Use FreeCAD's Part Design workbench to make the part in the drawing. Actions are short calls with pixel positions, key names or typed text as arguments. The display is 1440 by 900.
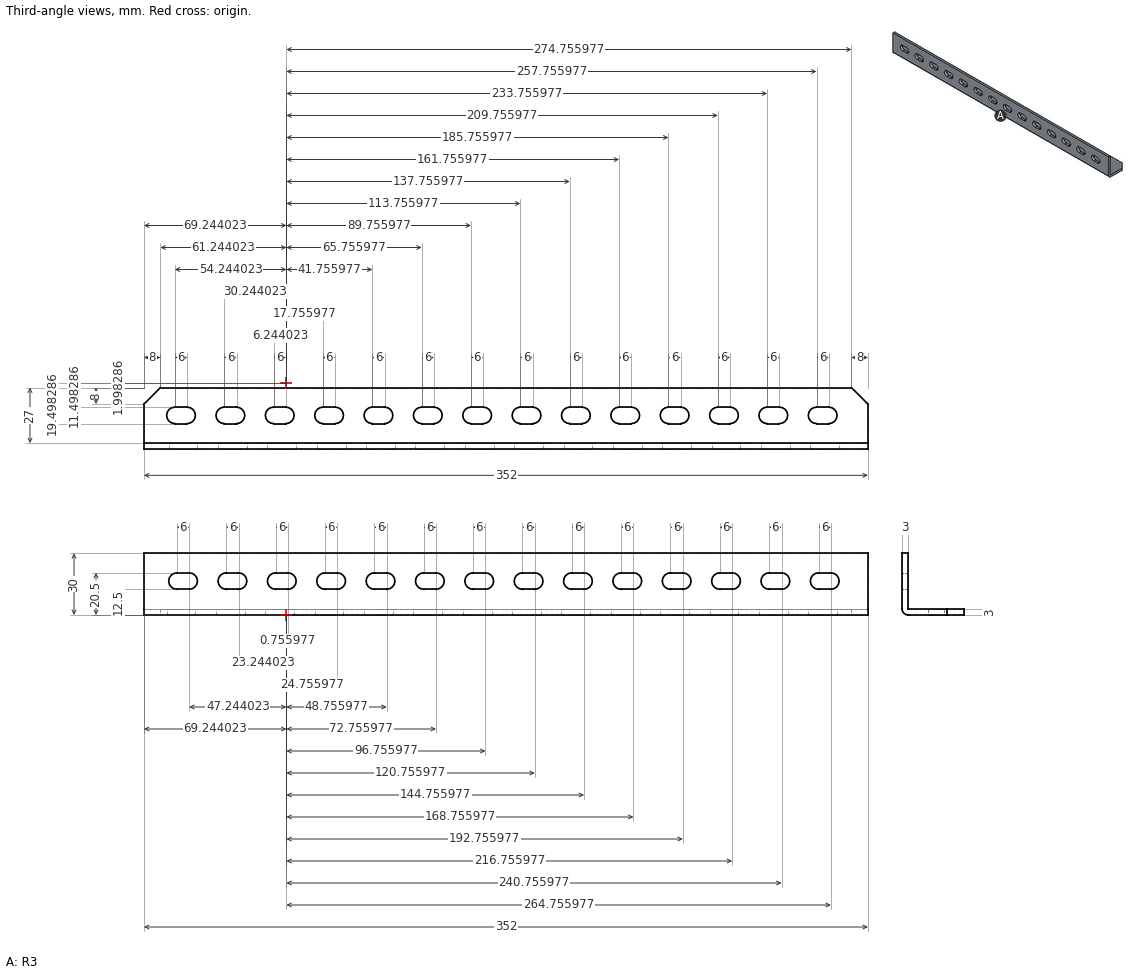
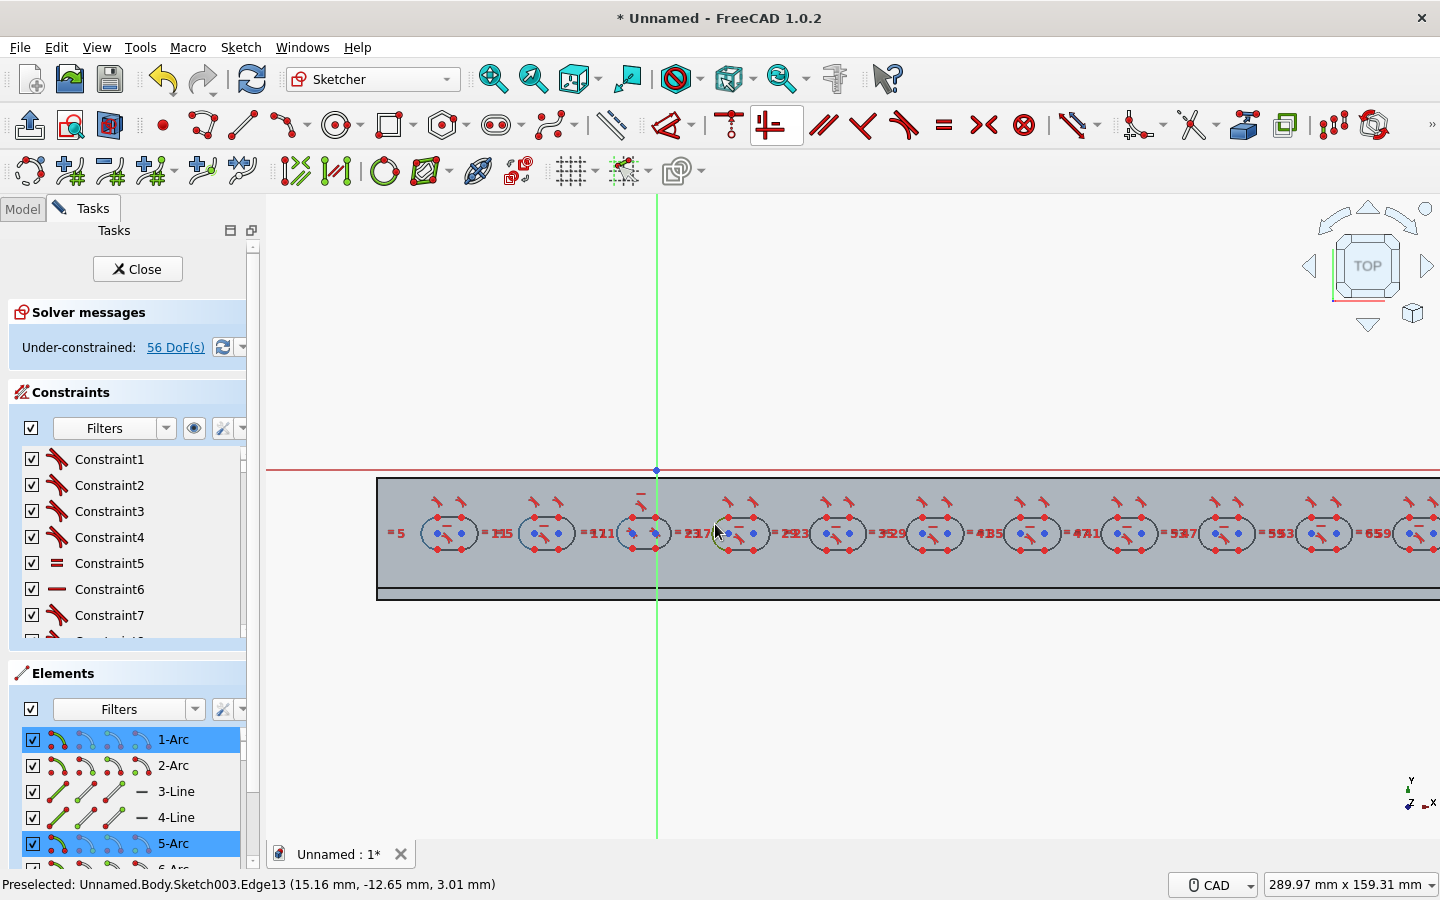
click(813, 524)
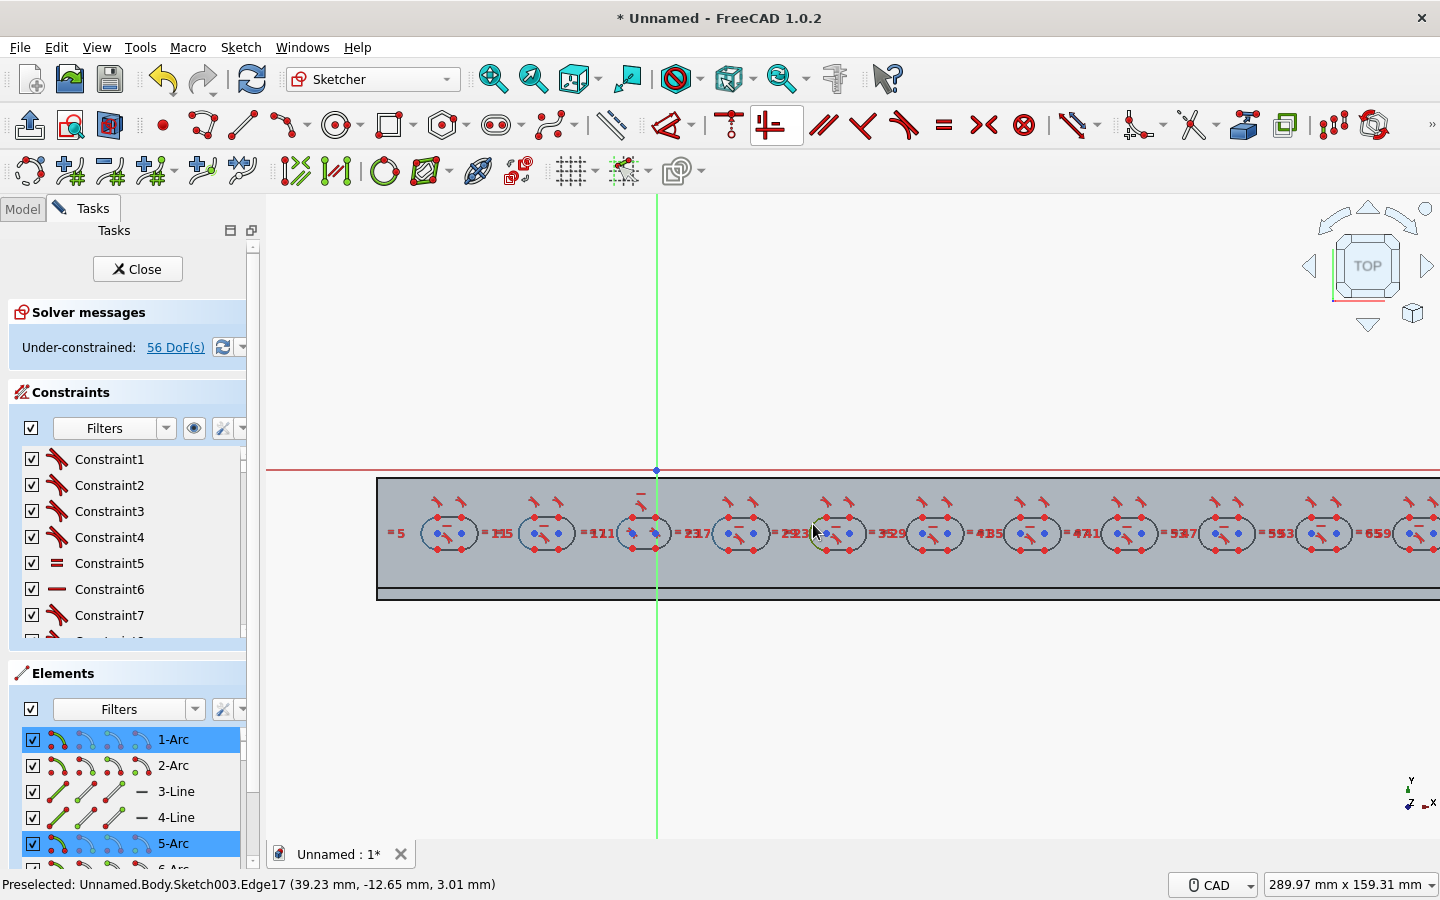
click(910, 524)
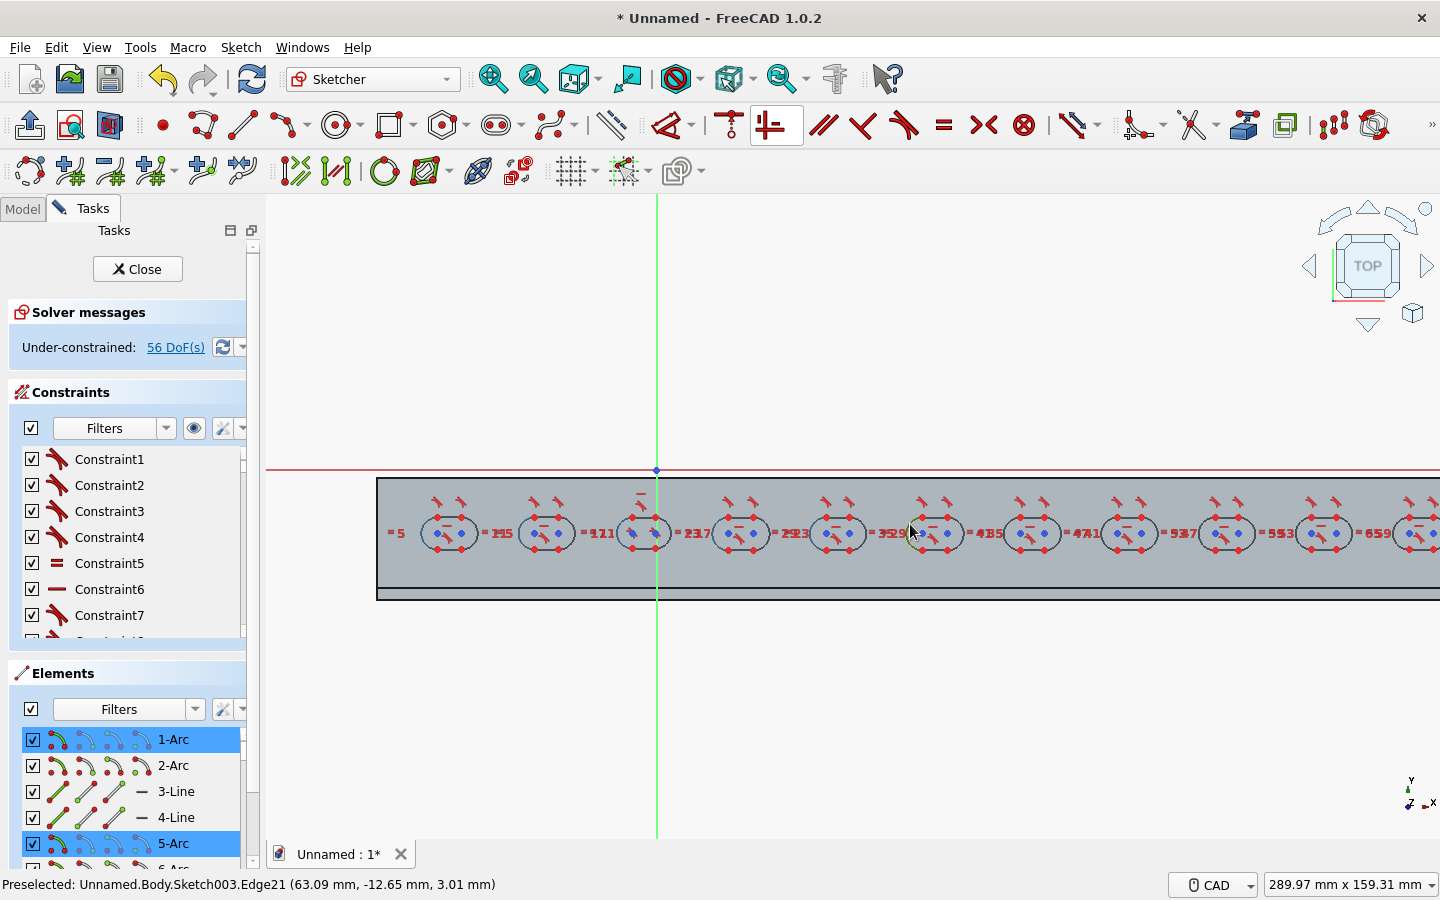
click(1007, 524)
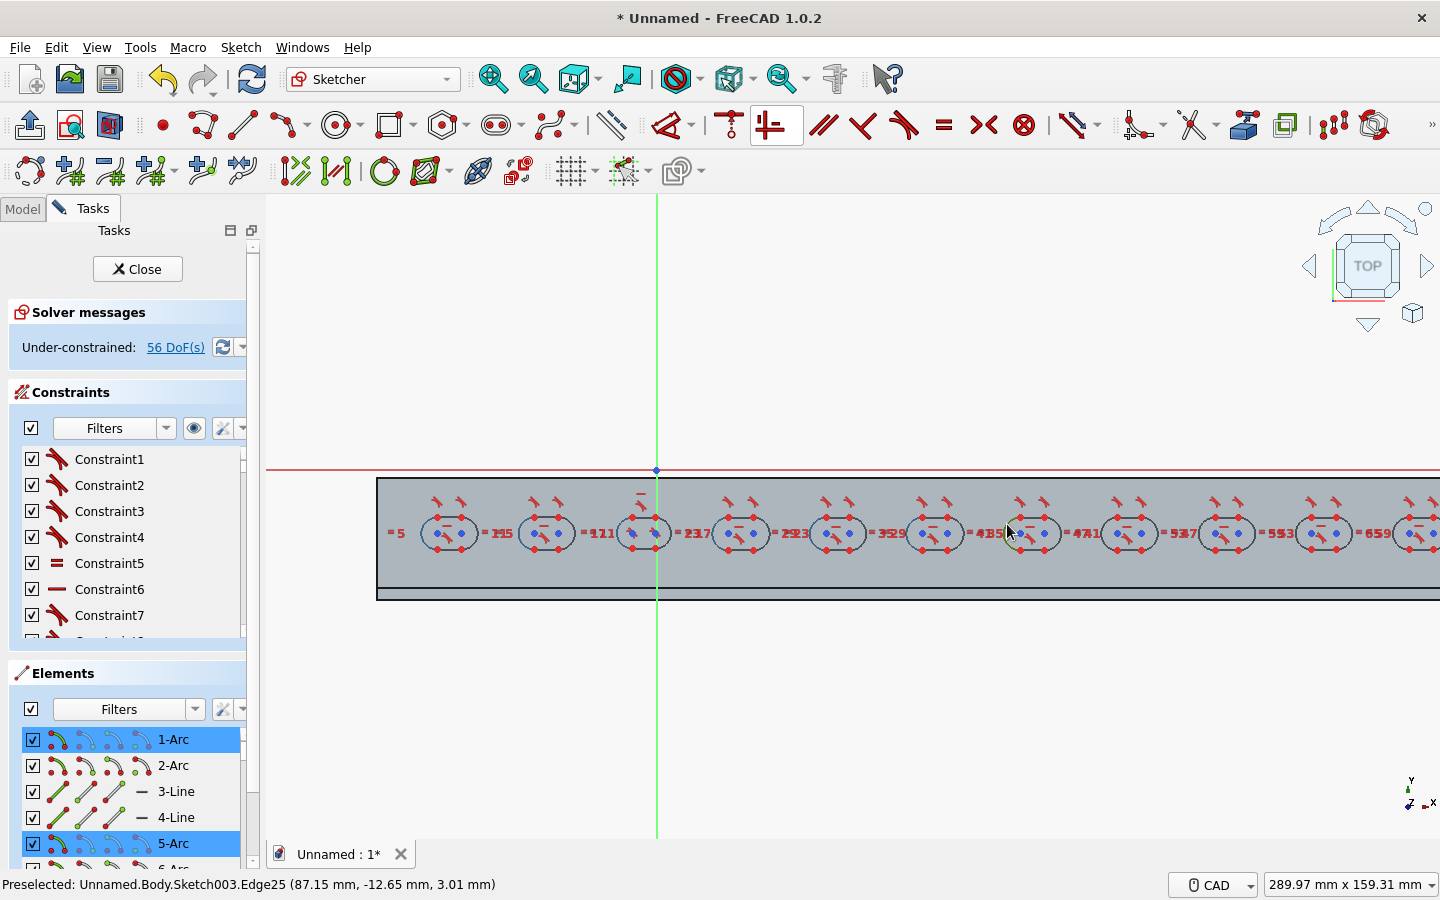
click(1104, 524)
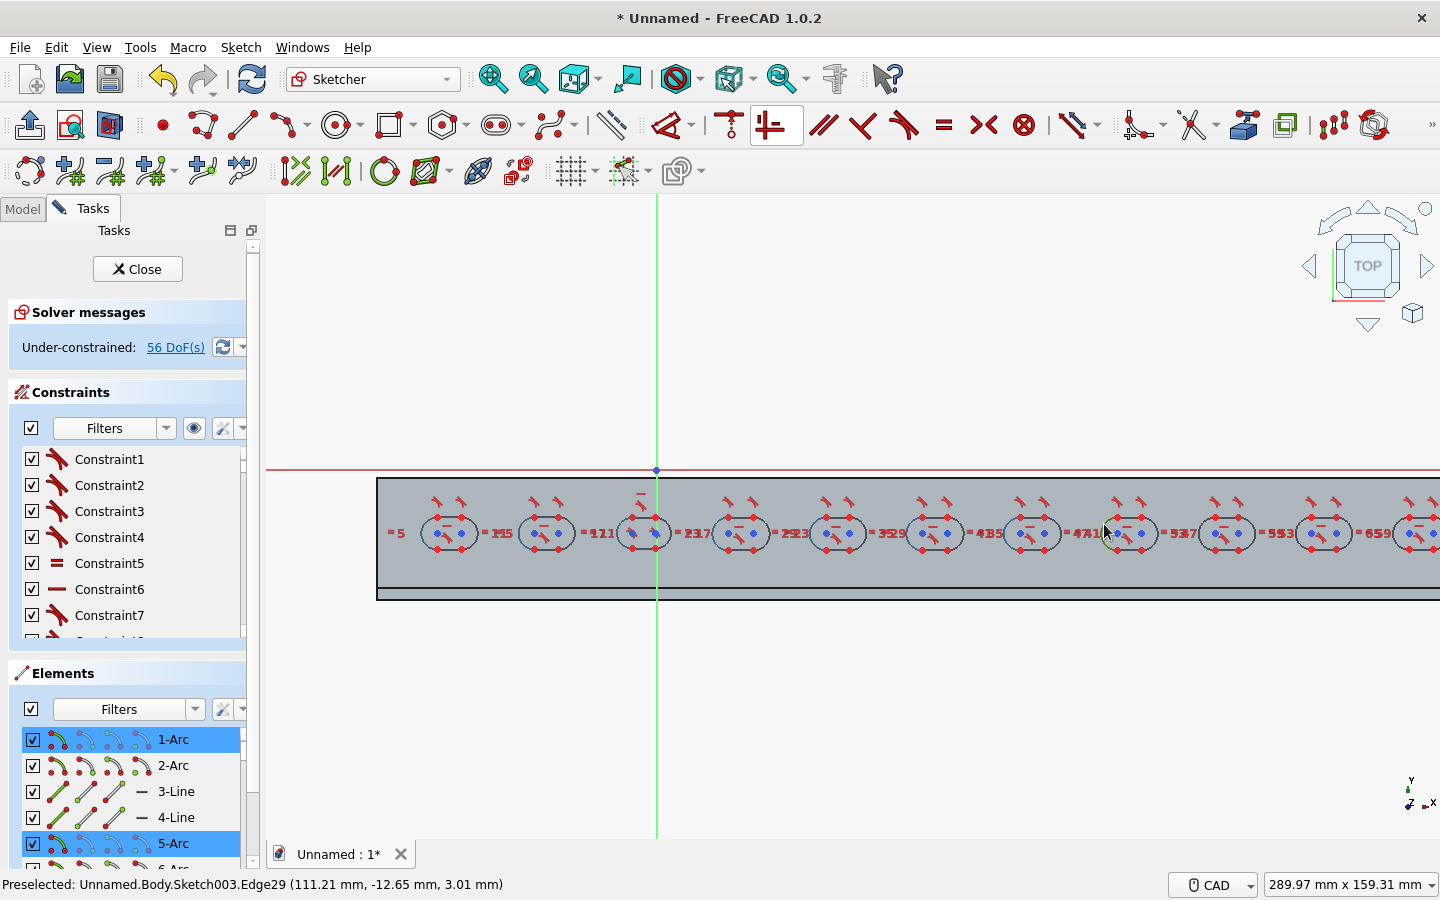
click(1202, 524)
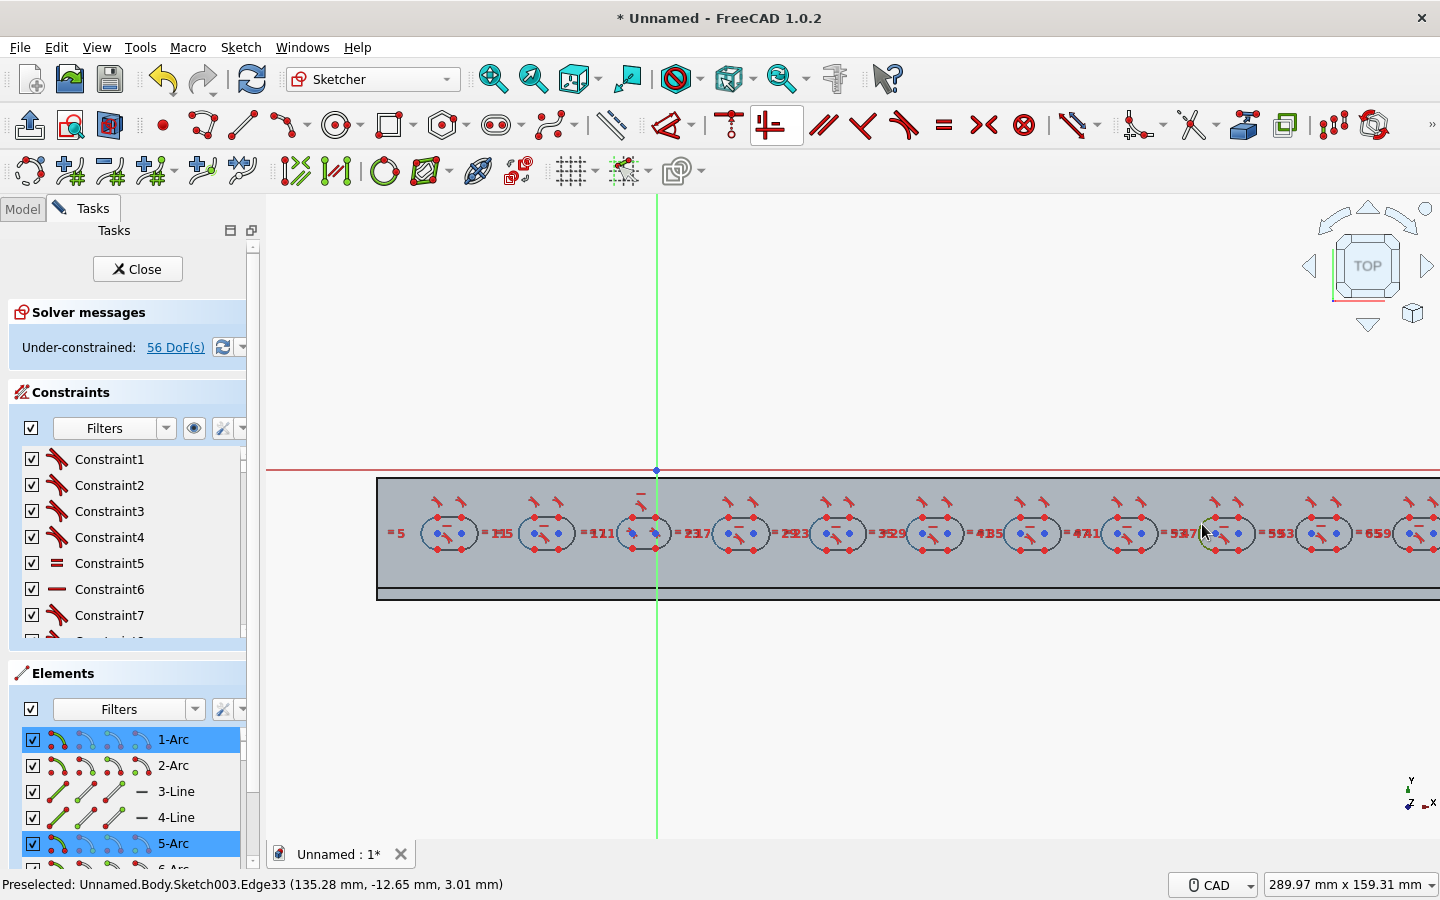
scroll(424, 525, down, 3)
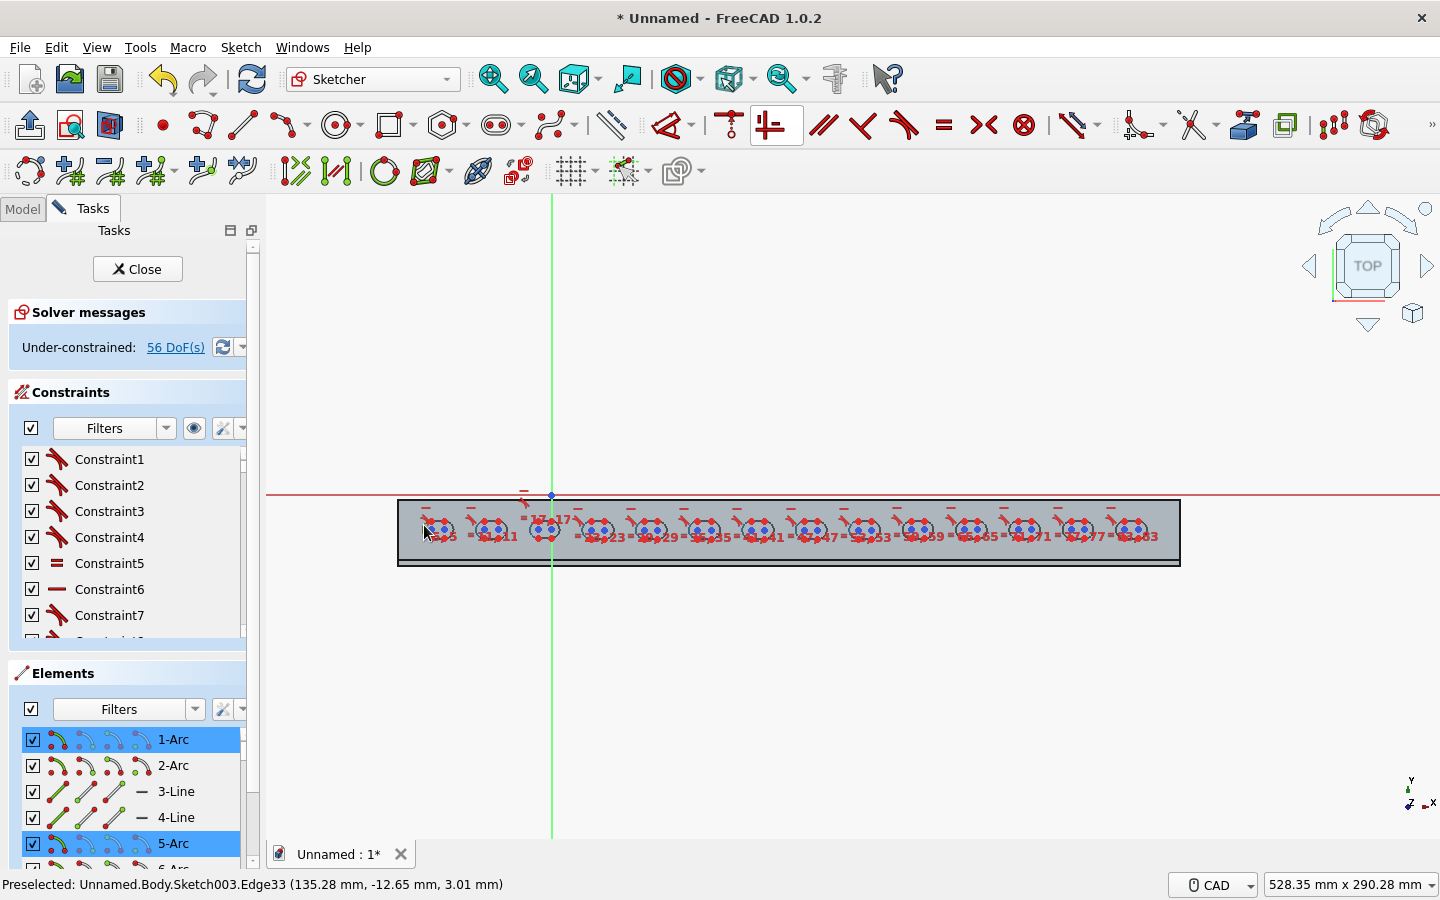
scroll(904, 525, up, 3)